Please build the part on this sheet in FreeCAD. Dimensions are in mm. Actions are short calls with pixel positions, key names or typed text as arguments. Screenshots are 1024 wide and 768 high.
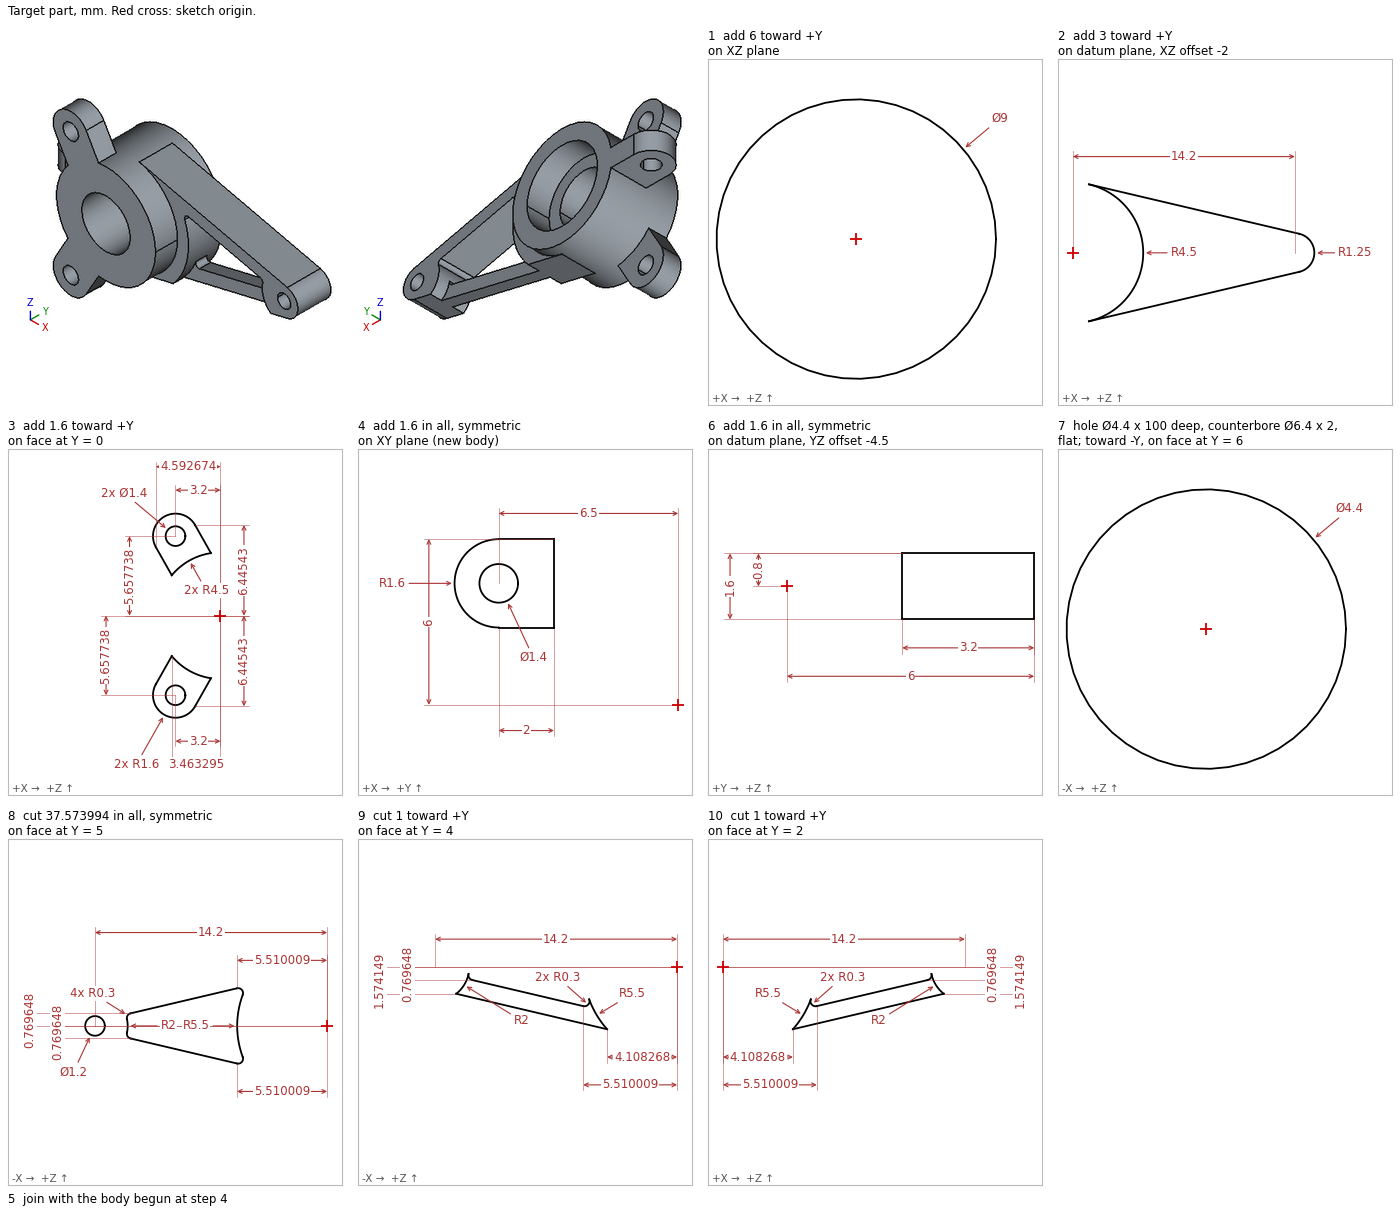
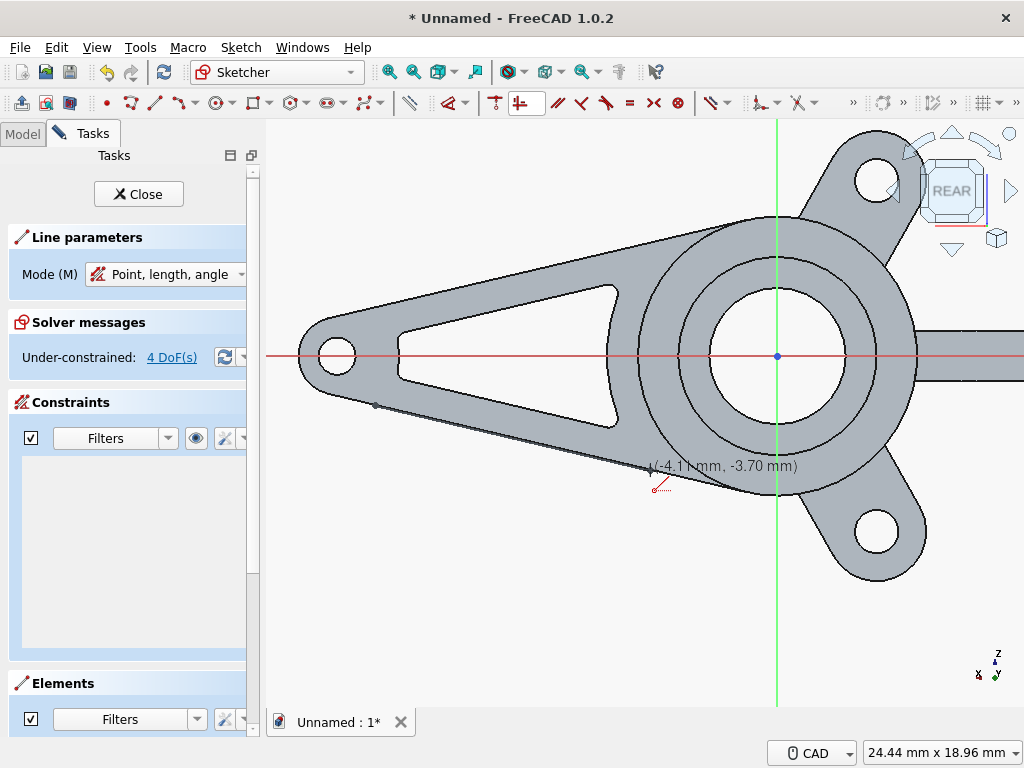
click(607, 427)
click(405, 380)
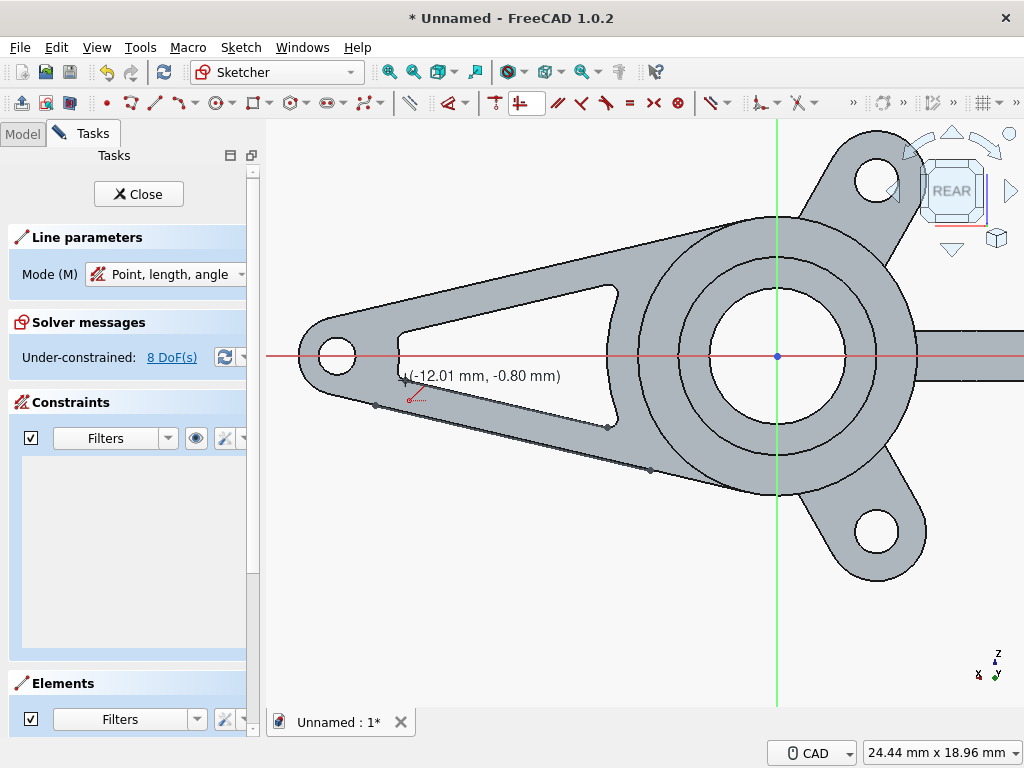
key(g)
key(3)
key(a)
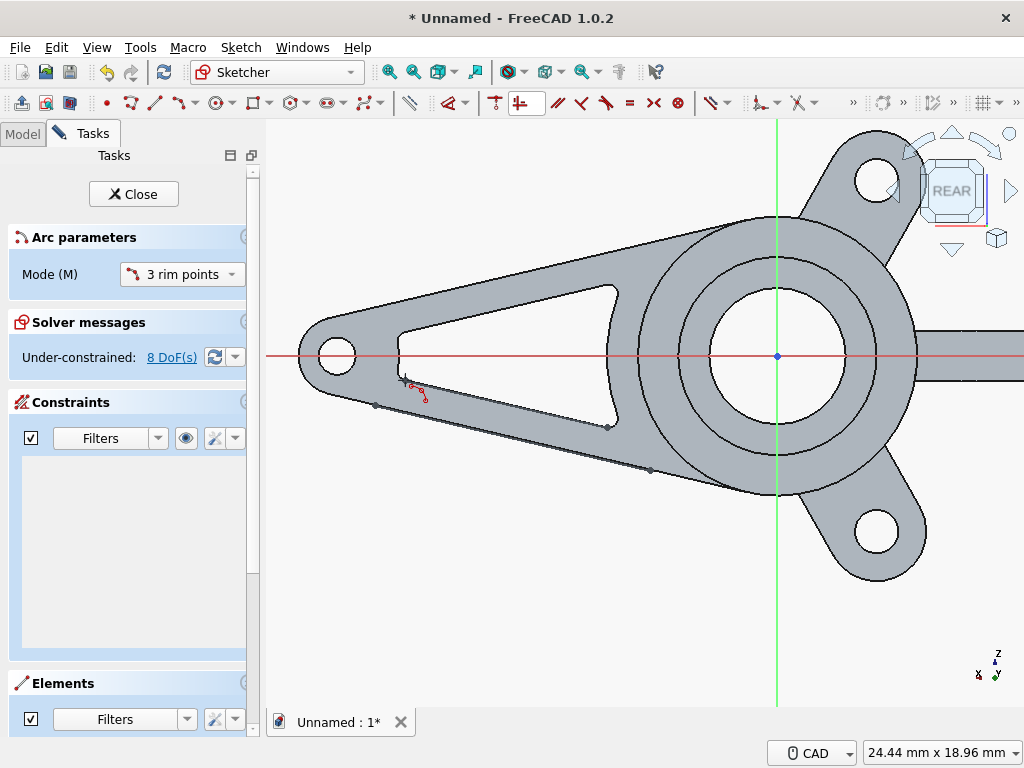
click(650, 471)
click(617, 415)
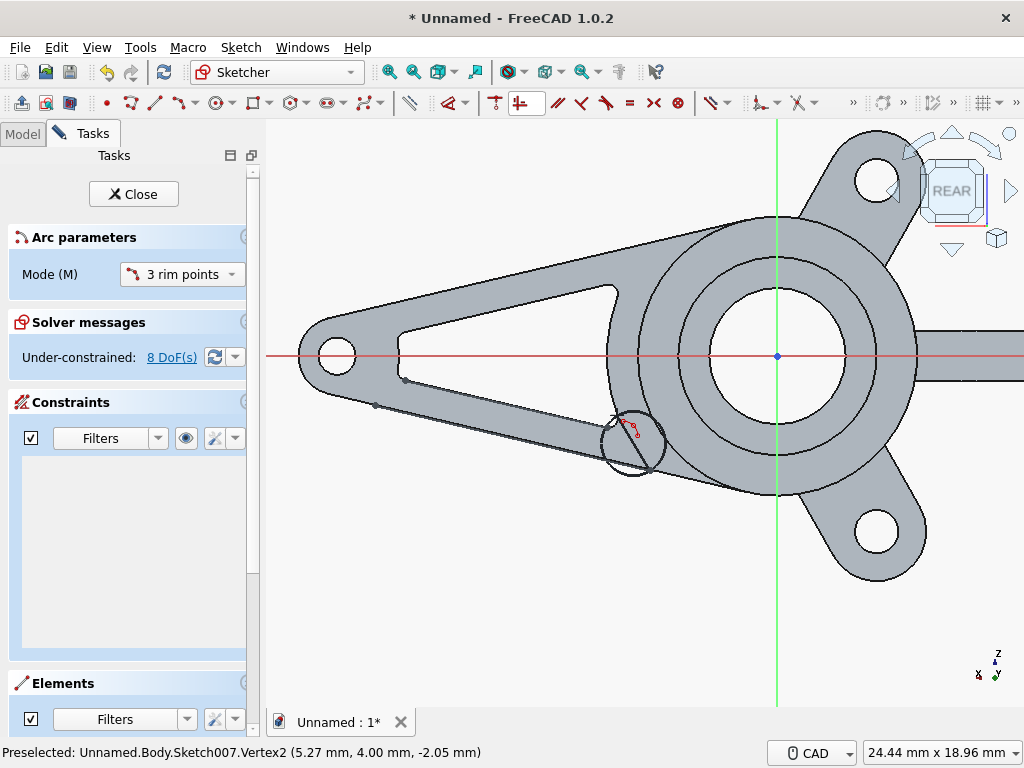
scroll(631, 444, up, 9)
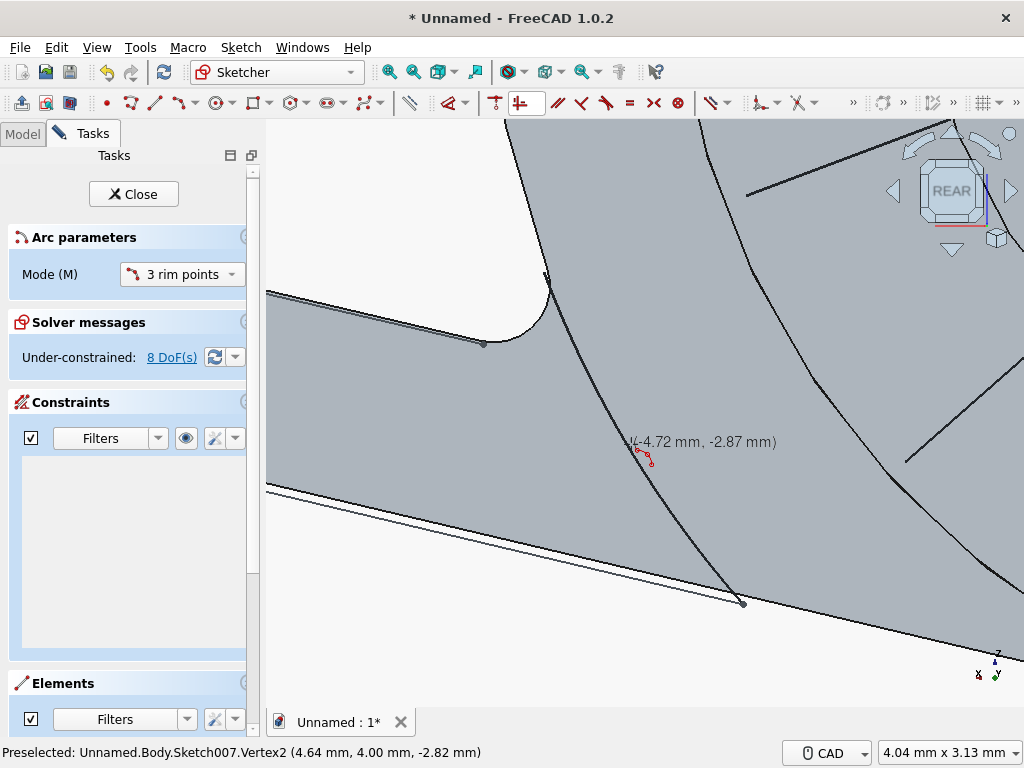
click(630, 440)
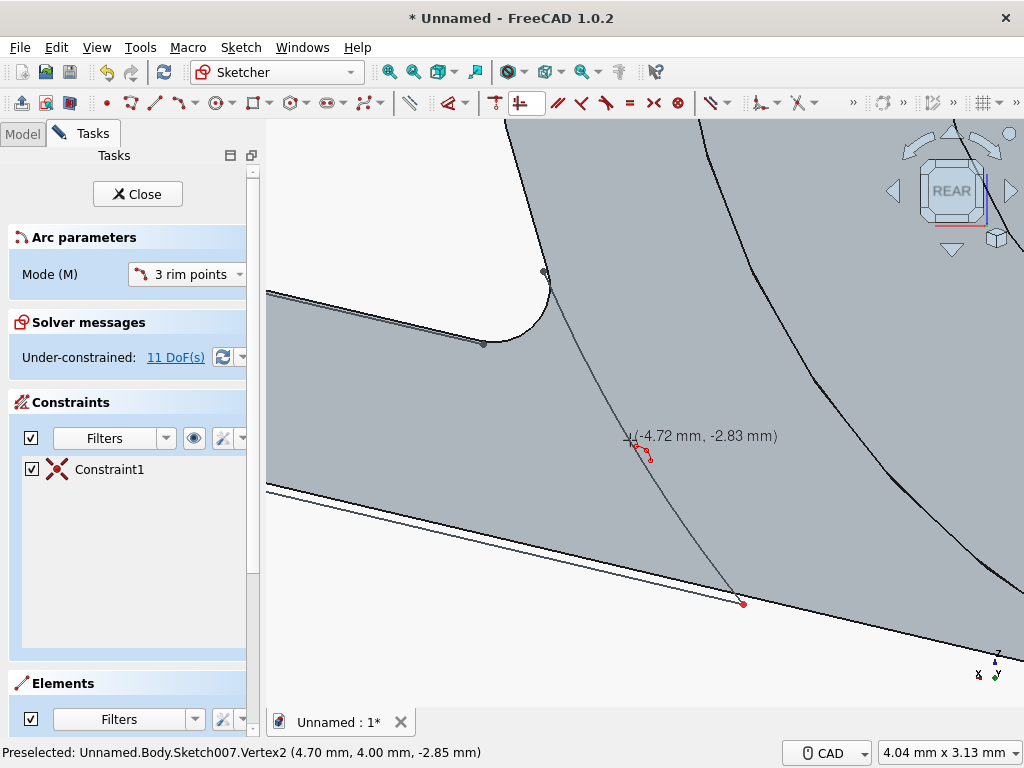
scroll(632, 445, down, 9)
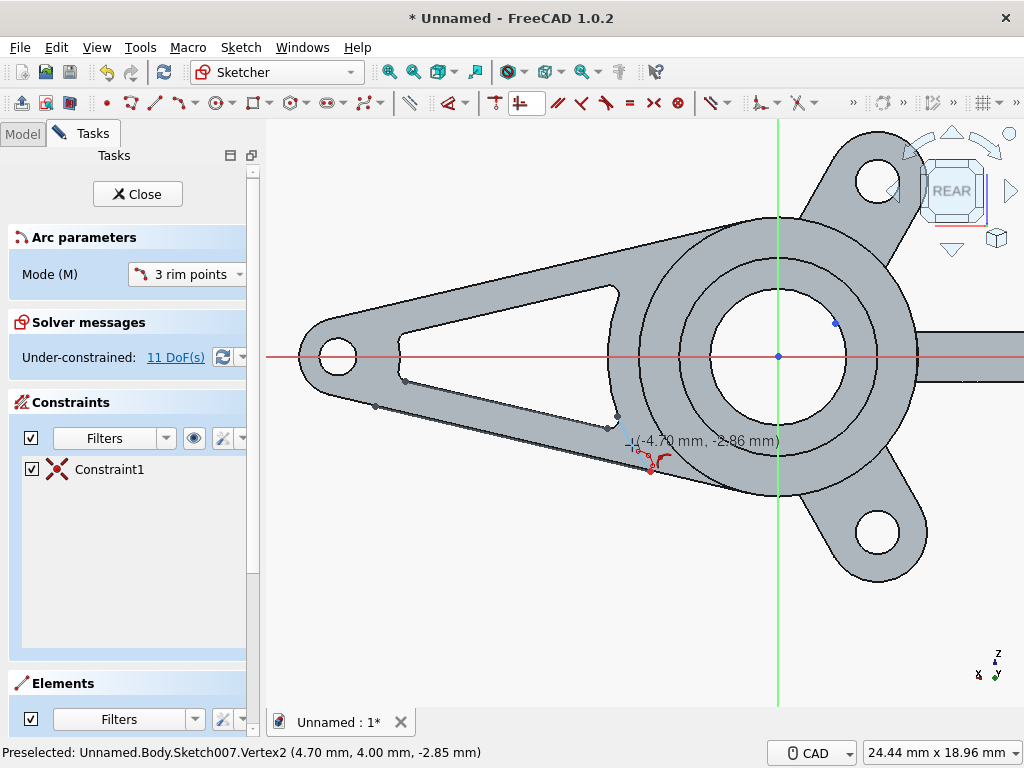
click(618, 417)
click(608, 429)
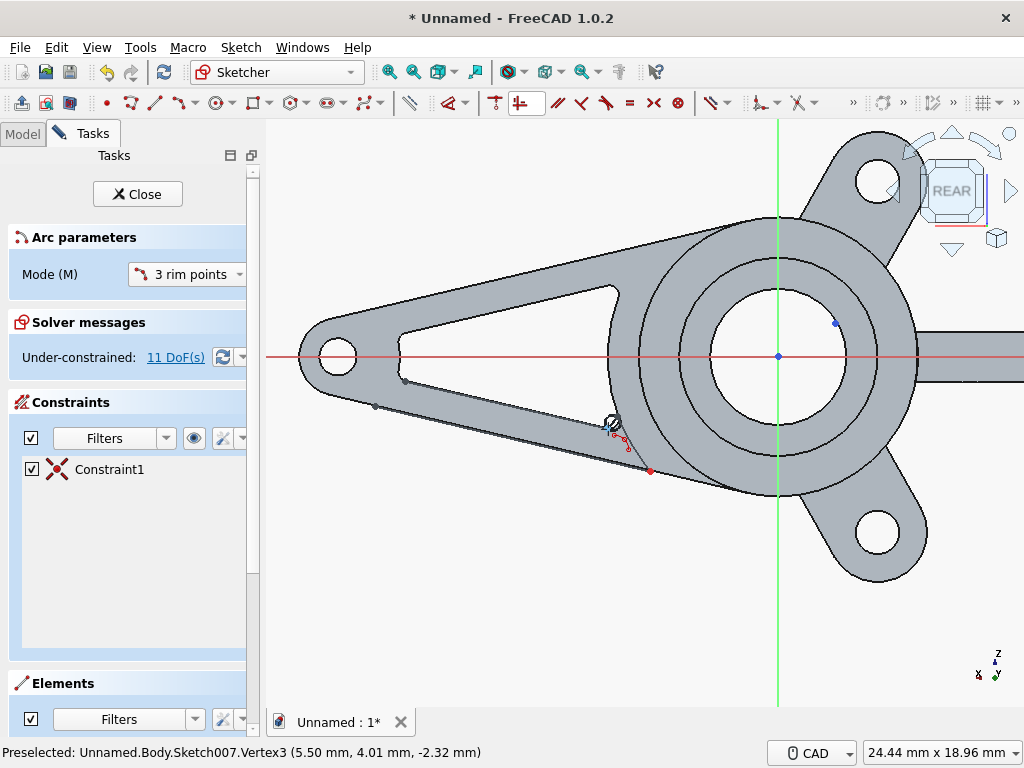
scroll(617, 425, up, 6)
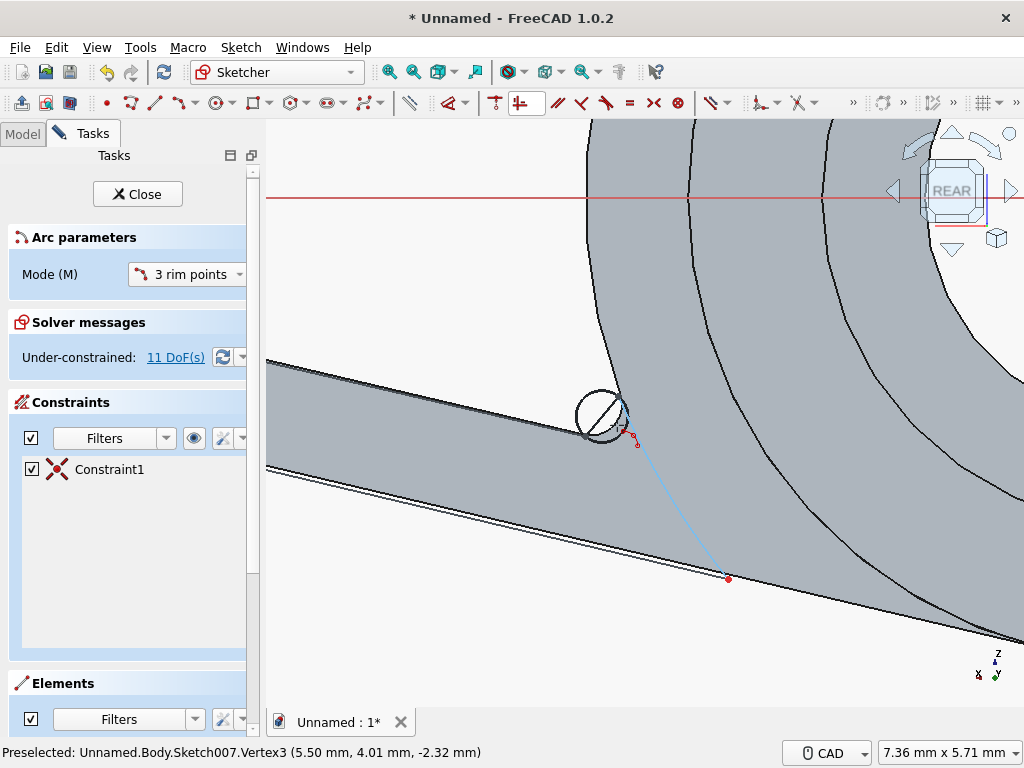
click(614, 425)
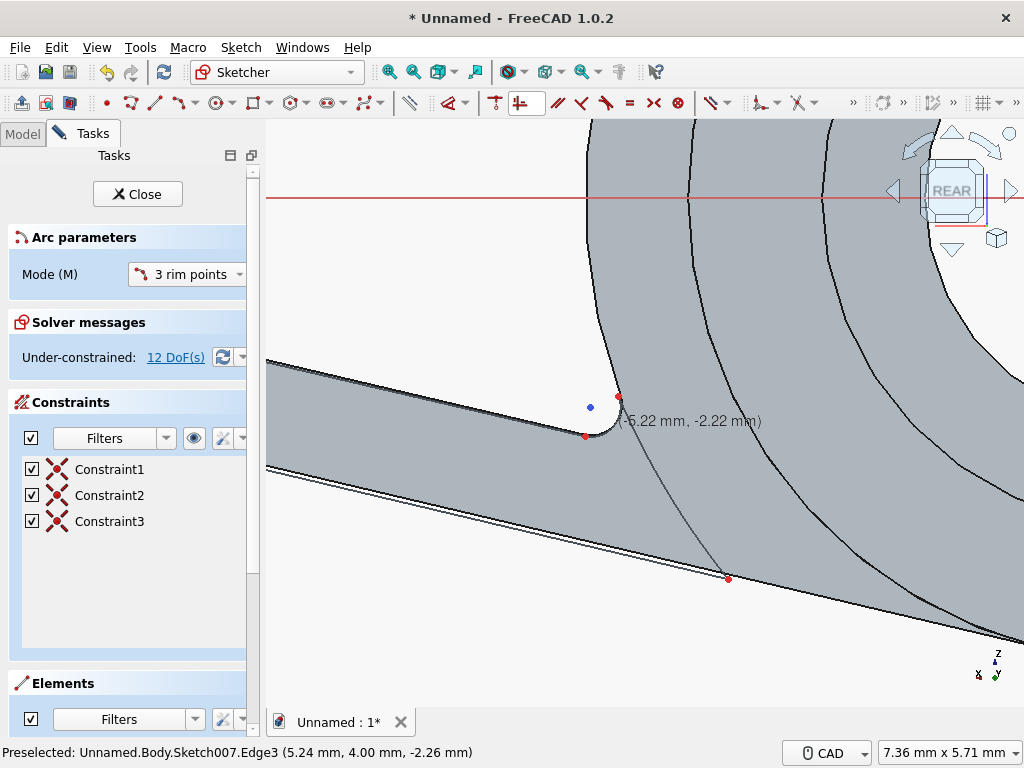
scroll(616, 425, down, 6)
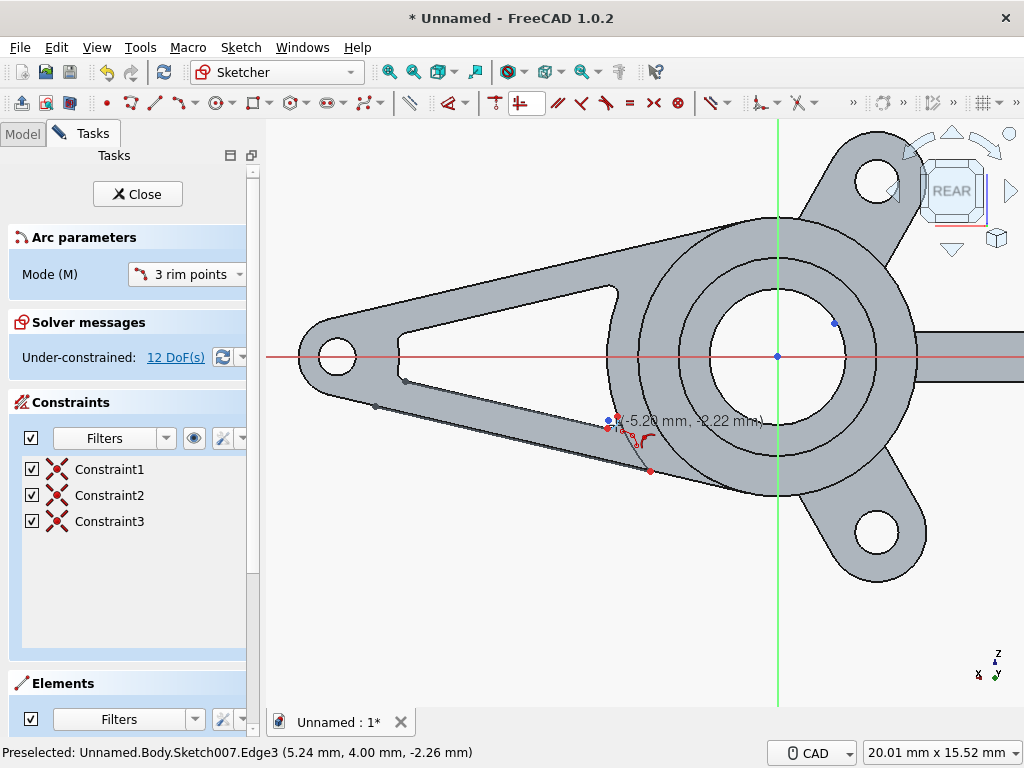
click(405, 382)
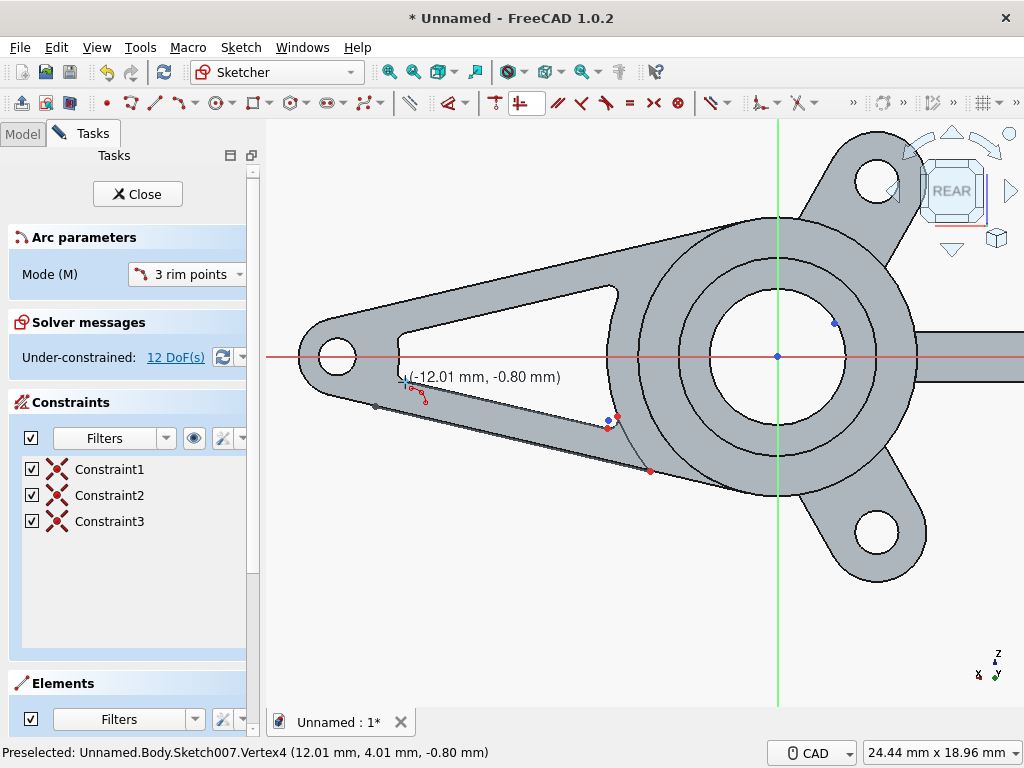
scroll(398, 370, up, 2)